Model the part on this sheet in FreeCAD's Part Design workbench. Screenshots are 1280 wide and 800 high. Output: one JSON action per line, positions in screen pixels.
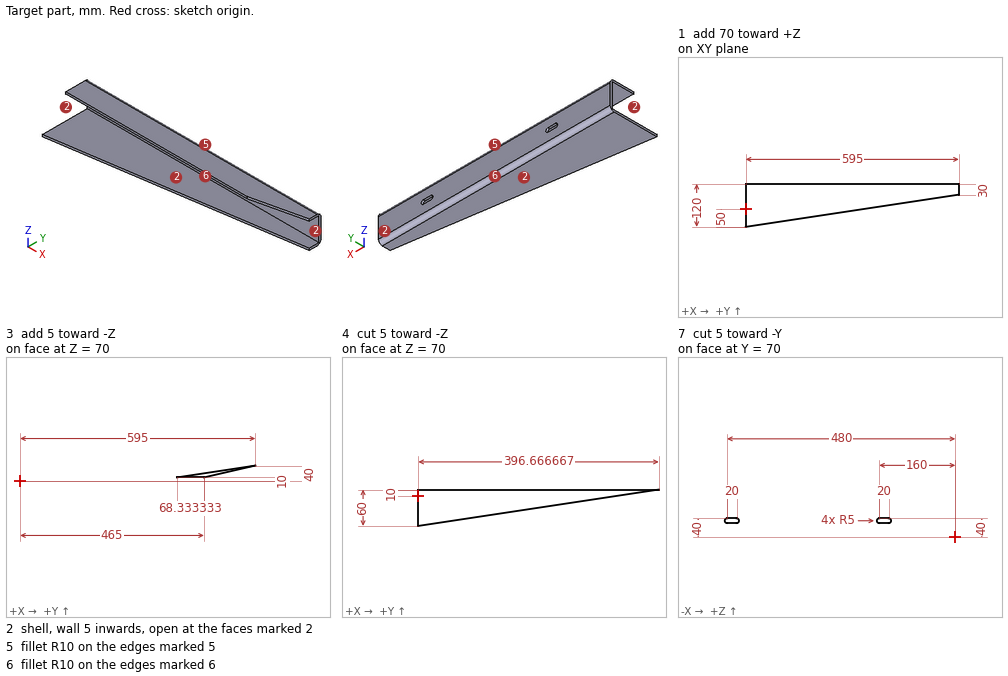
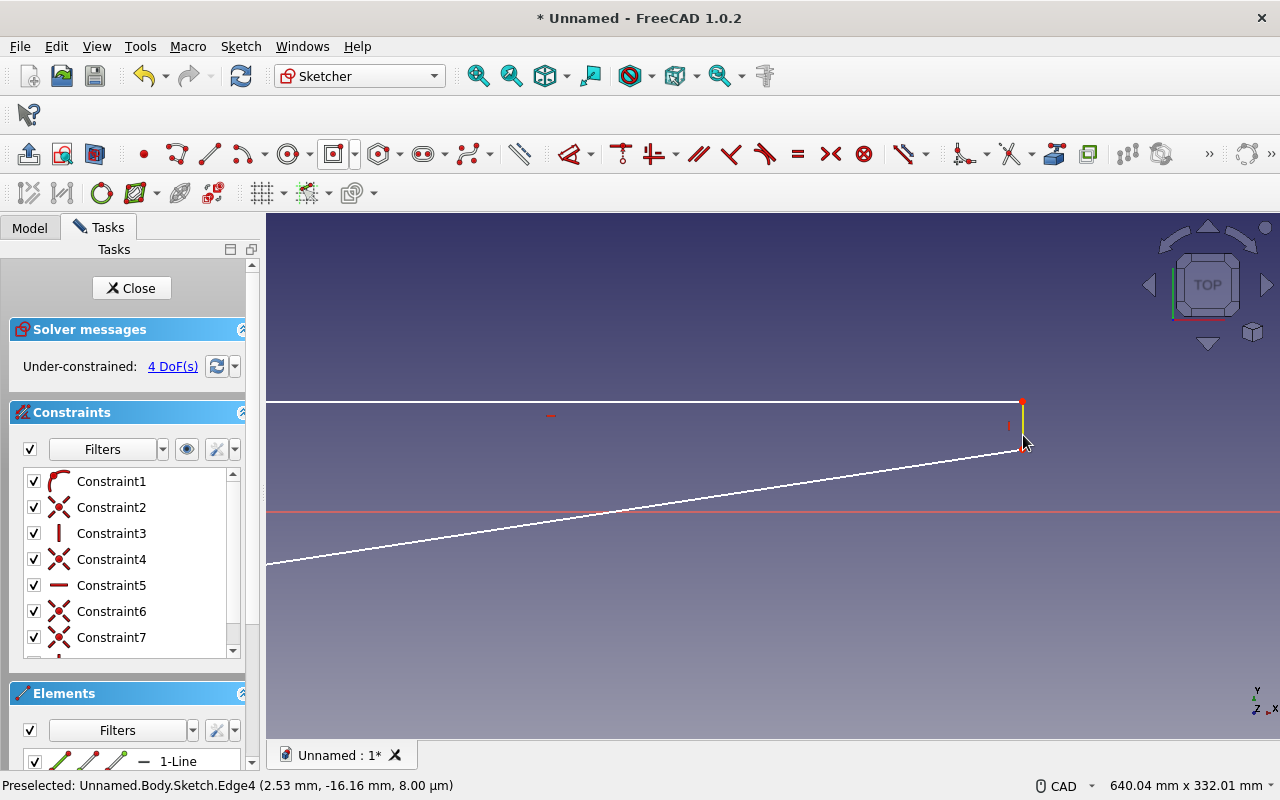
{"action": "left_click", "coordinate": [1023, 435]}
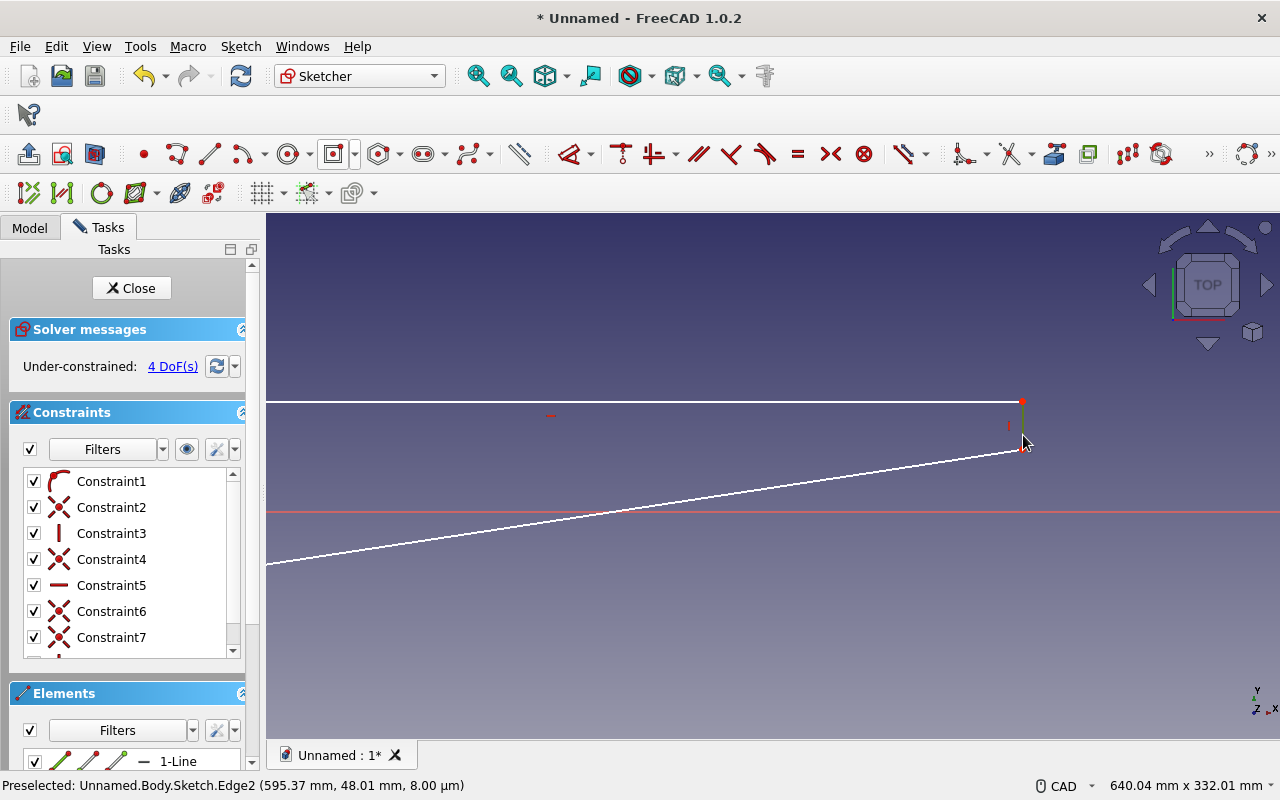
{"action": "left_click", "coordinate": [590, 154]}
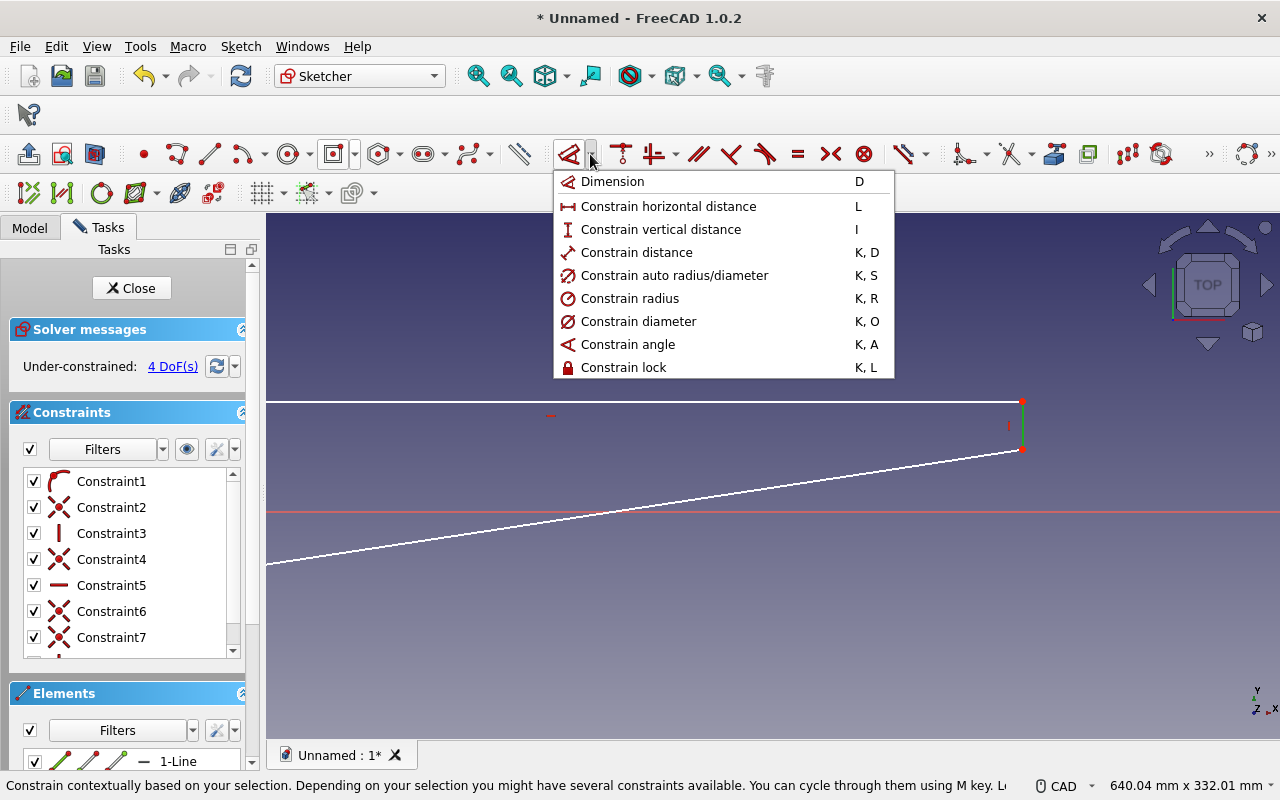
{"action": "left_click", "coordinate": [724, 230]}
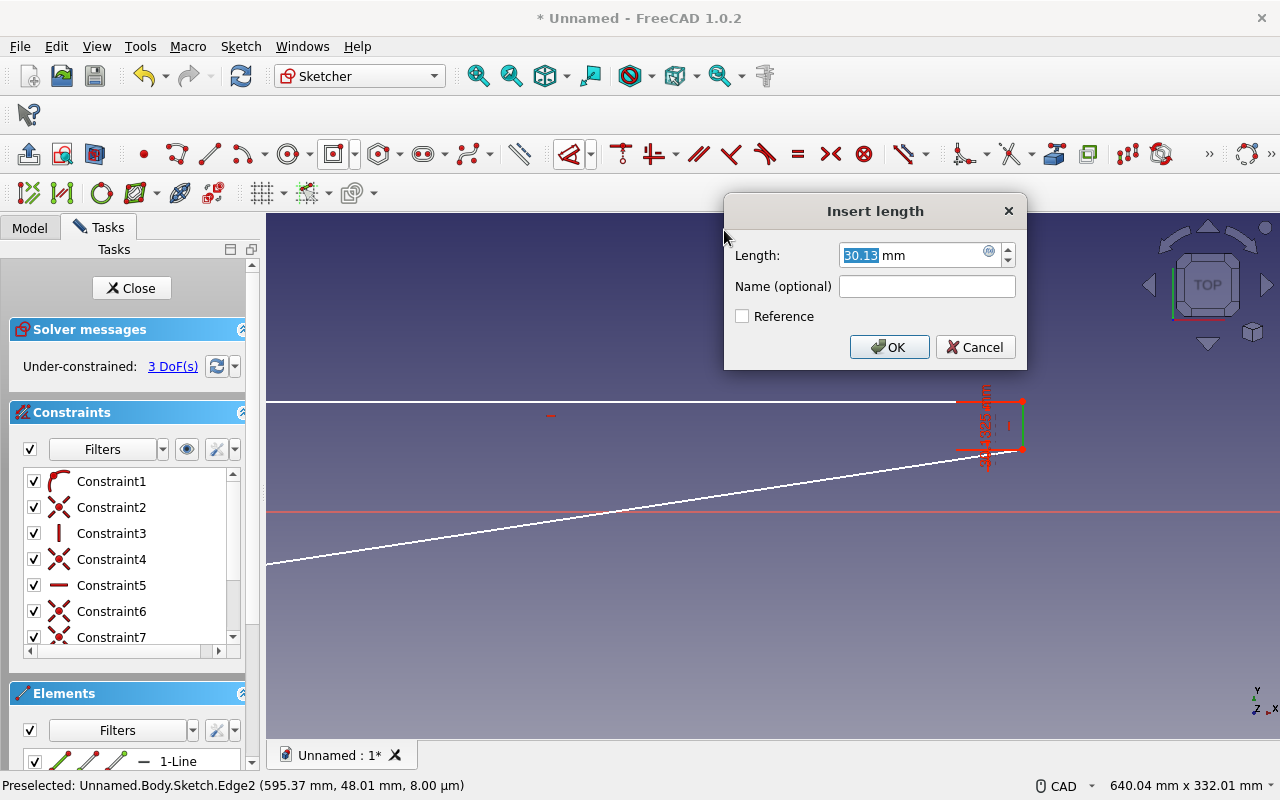
{"action": "type", "text": "30"}
{"action": "key", "text": "Return"}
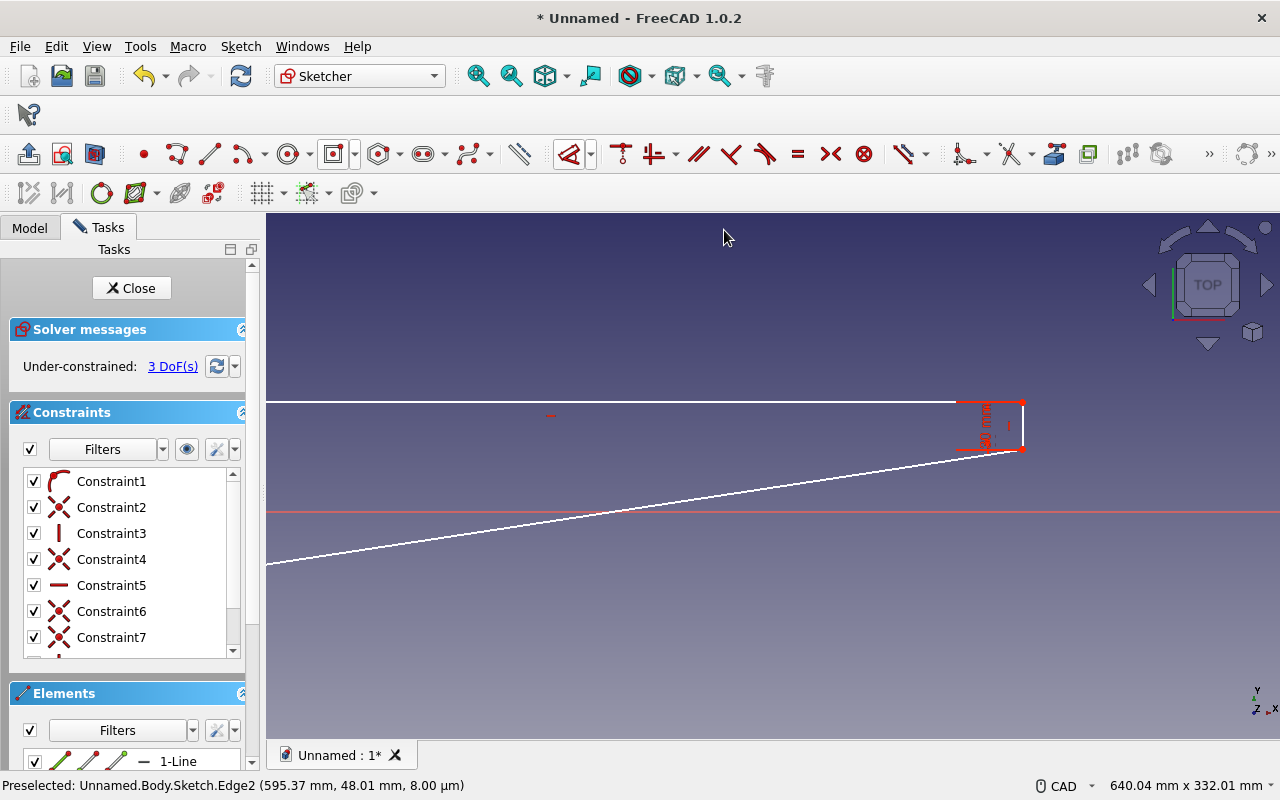
{"action": "left_click", "coordinate": [740, 402]}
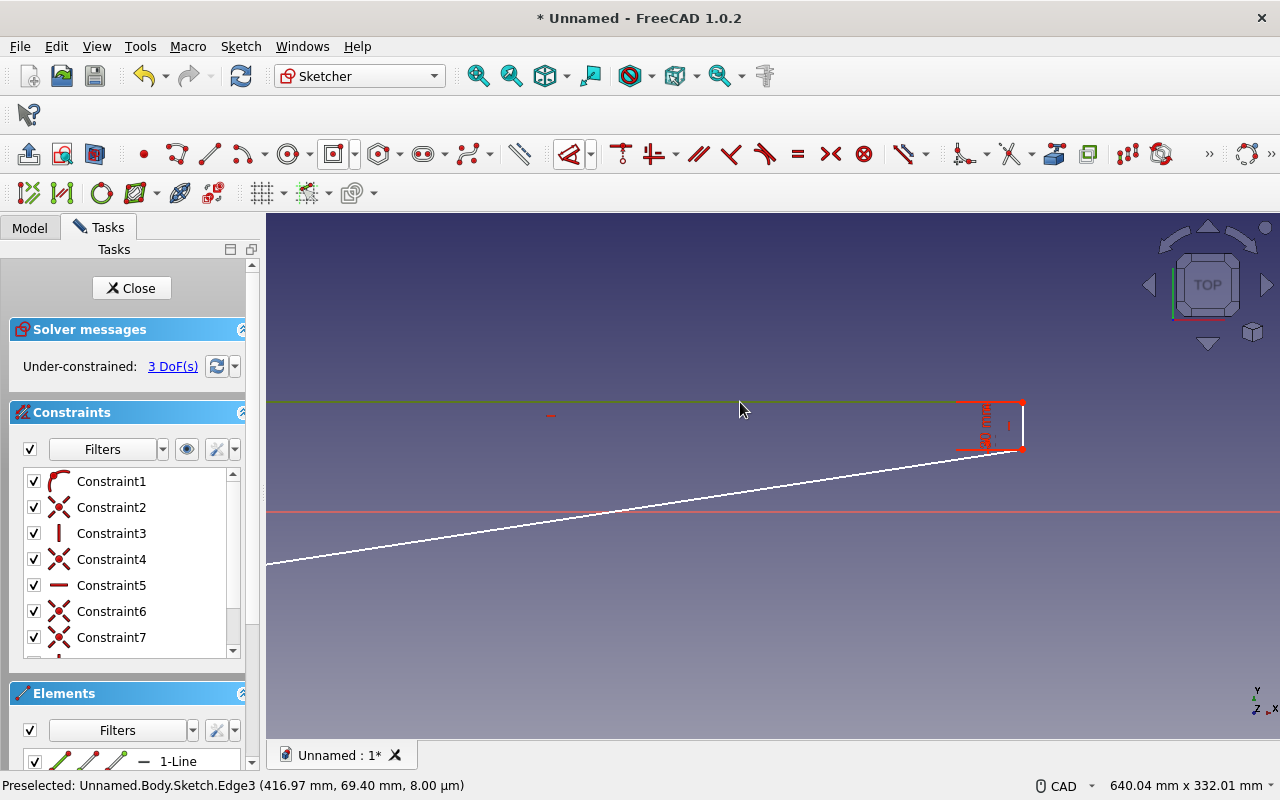
{"action": "left_click", "coordinate": [590, 154]}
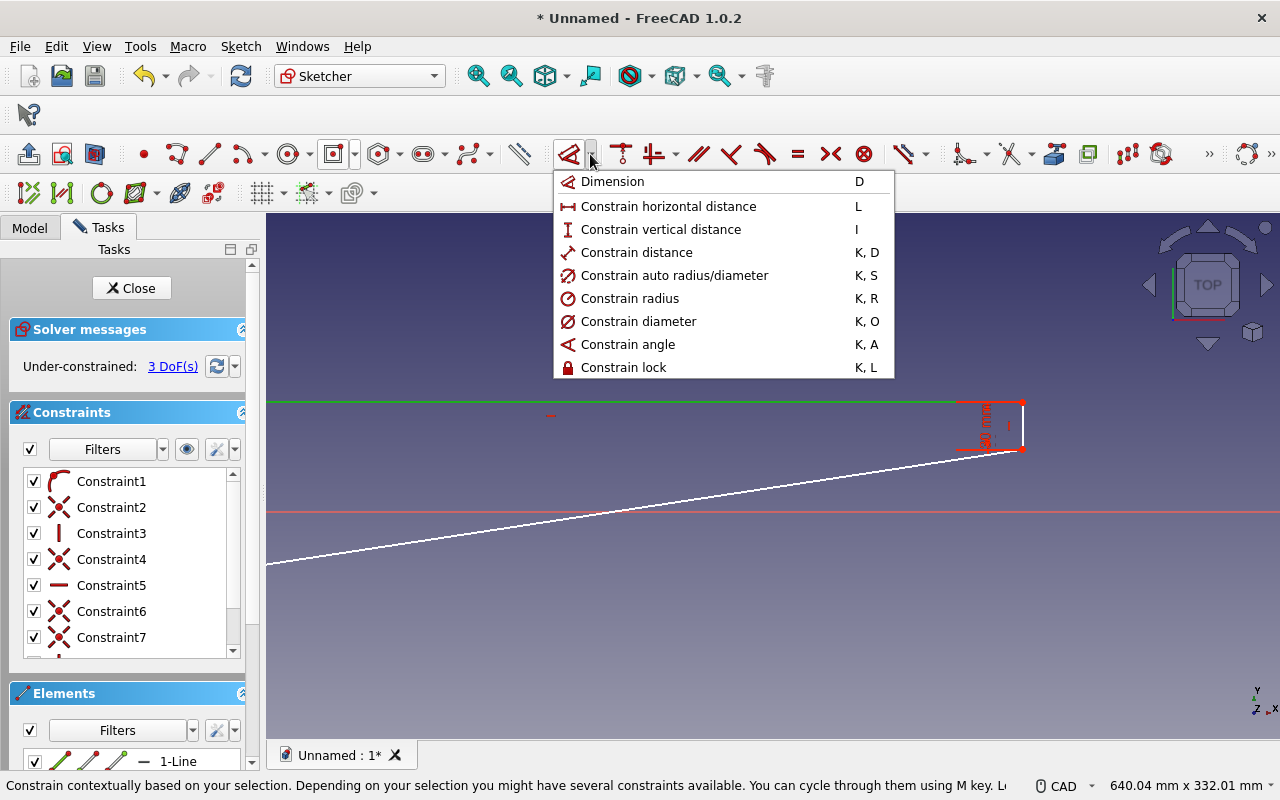
{"action": "left_click", "coordinate": [724, 206]}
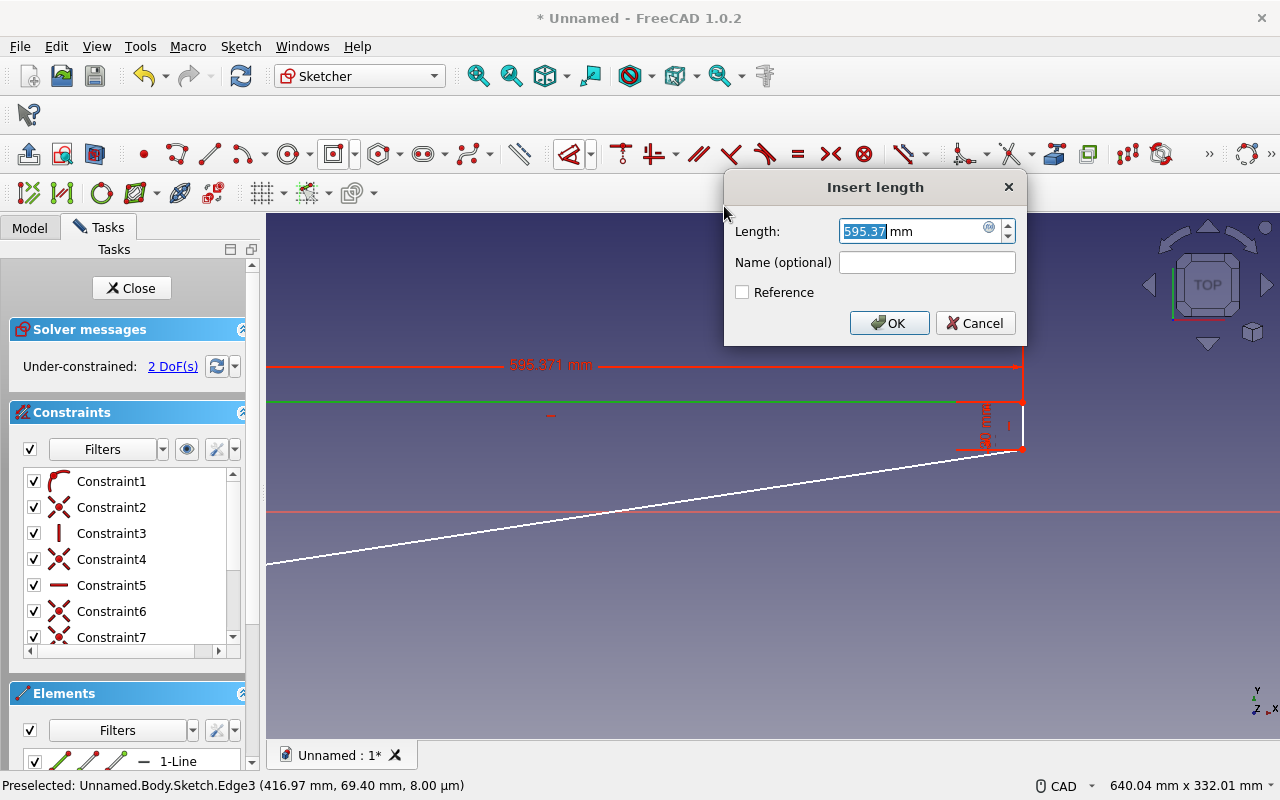
{"action": "type", "text": "595"}
{"action": "key", "text": "Return"}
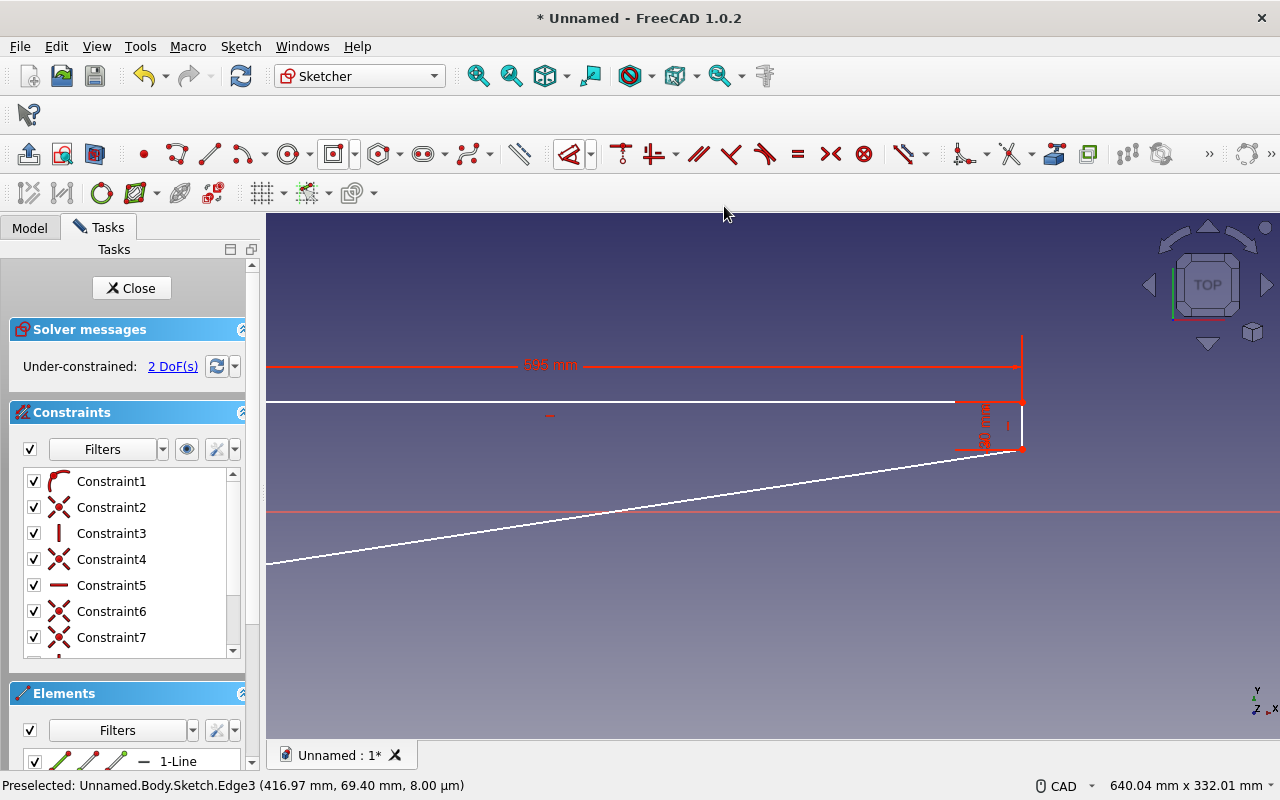
{"action": "scroll", "coordinate": [1017, 435], "scroll_direction": "down", "scroll_amount": 2}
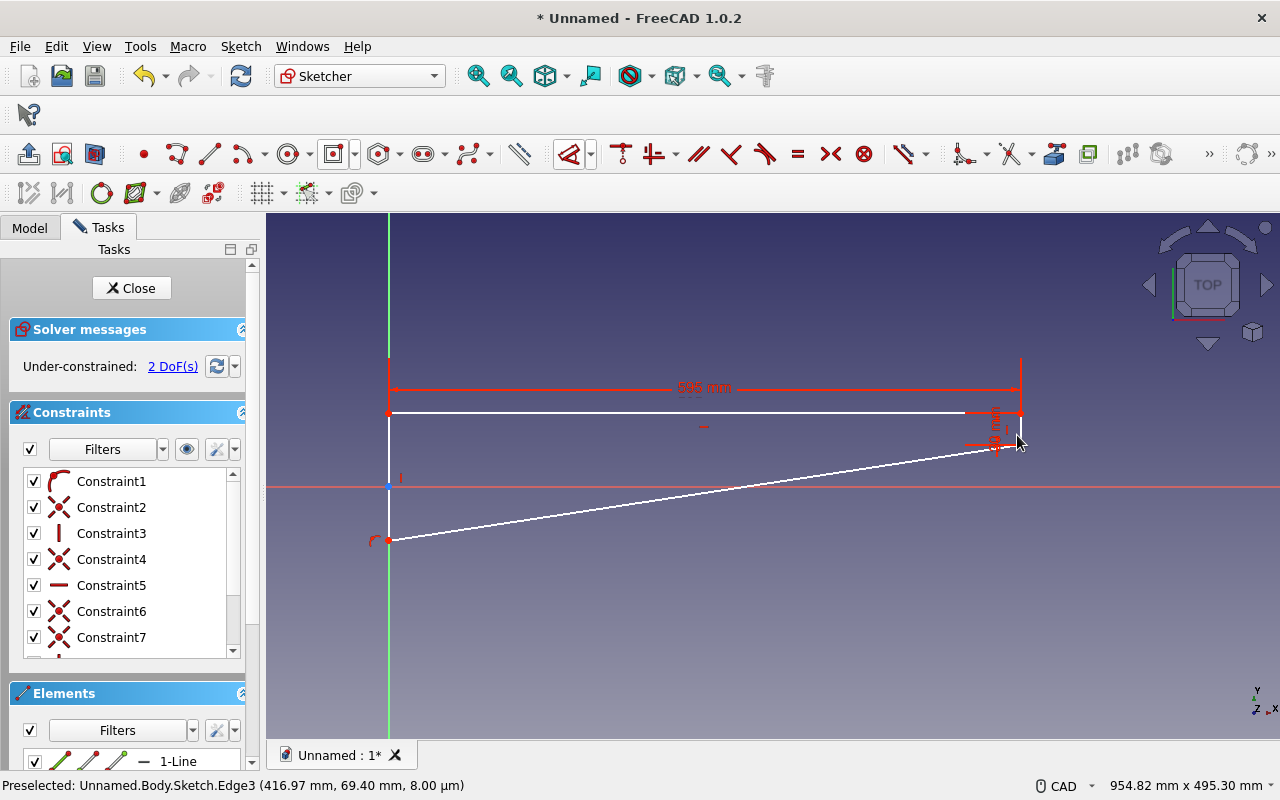
{"action": "left_click", "coordinate": [389, 451]}